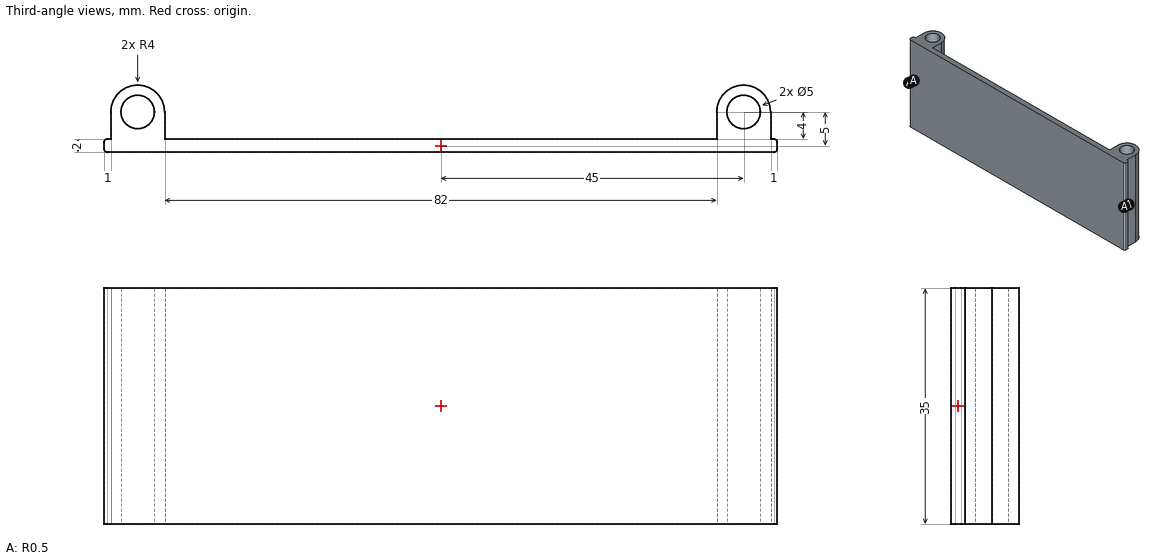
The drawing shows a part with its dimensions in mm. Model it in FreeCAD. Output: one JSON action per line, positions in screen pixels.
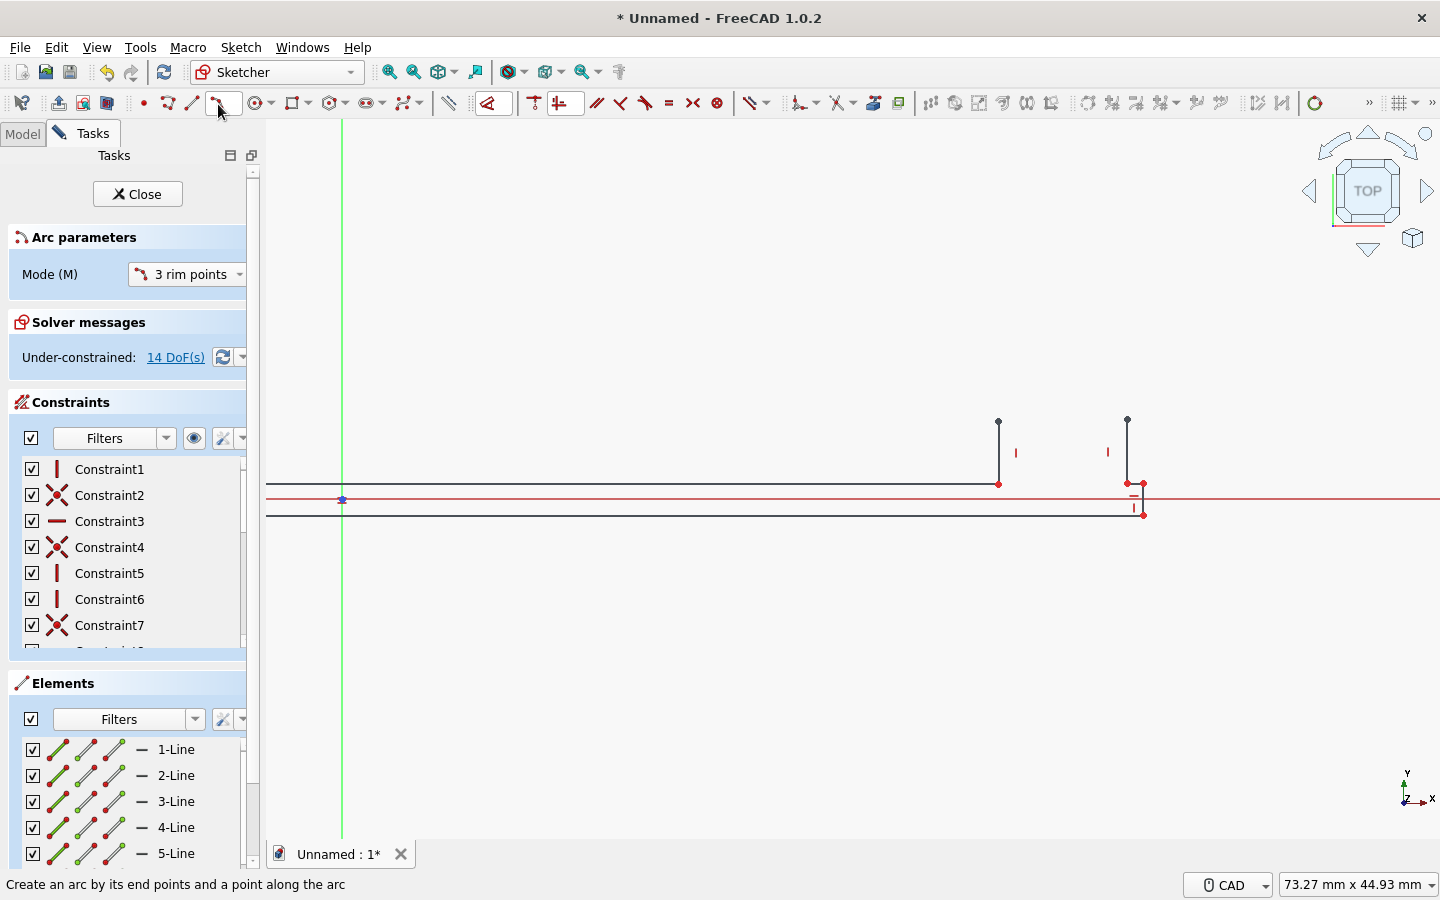
{"action": "scroll", "coordinate": [1145, 515], "scroll_direction": "down", "scroll_amount": 4}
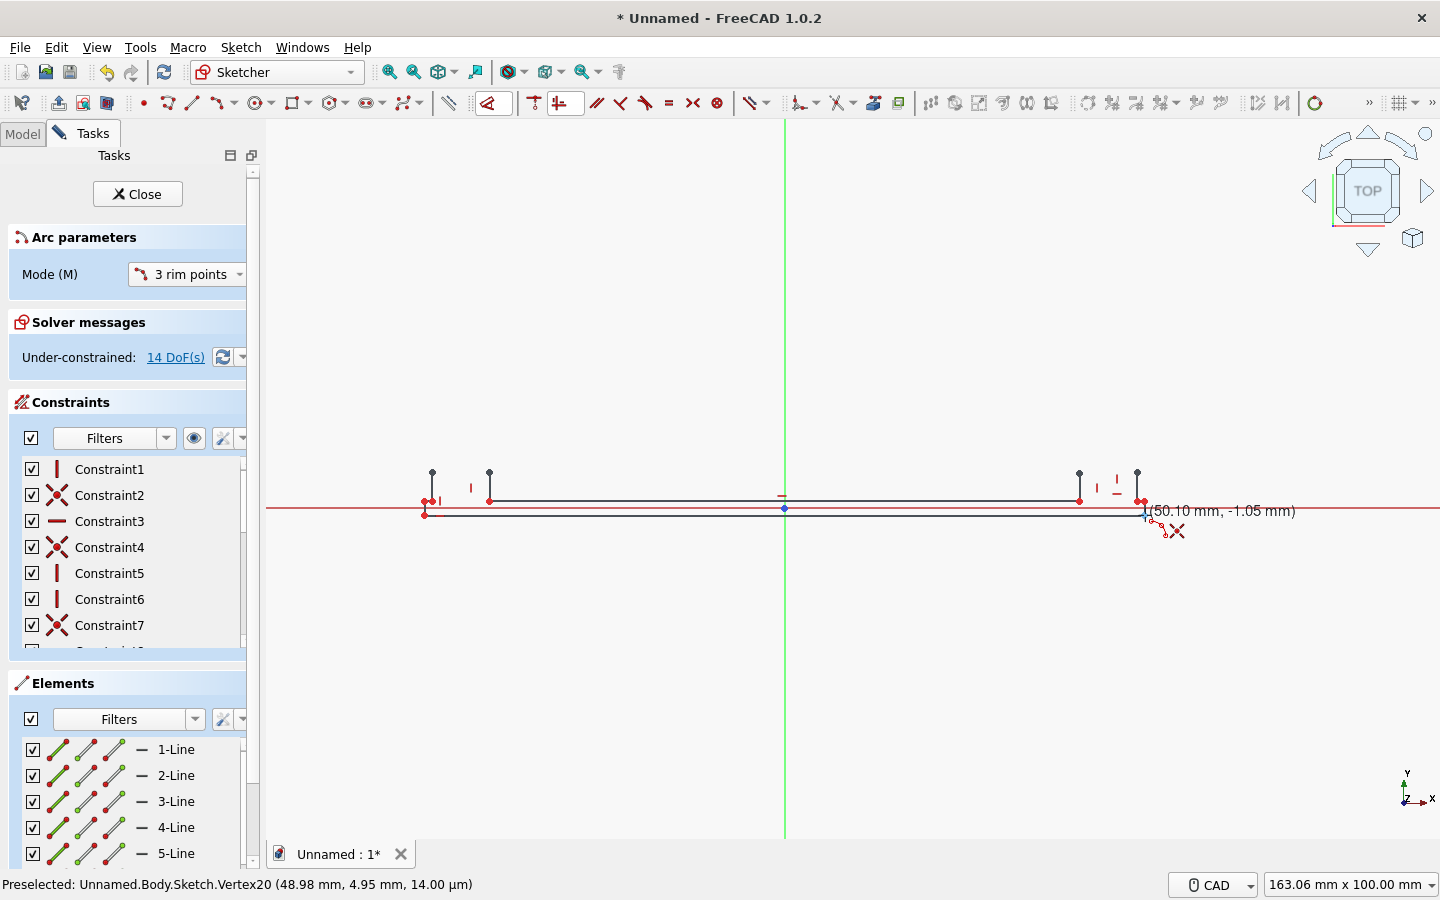
{"action": "left_click", "coordinate": [490, 473]}
{"action": "left_click", "coordinate": [432, 473]}
{"action": "left_click", "coordinate": [461, 443]}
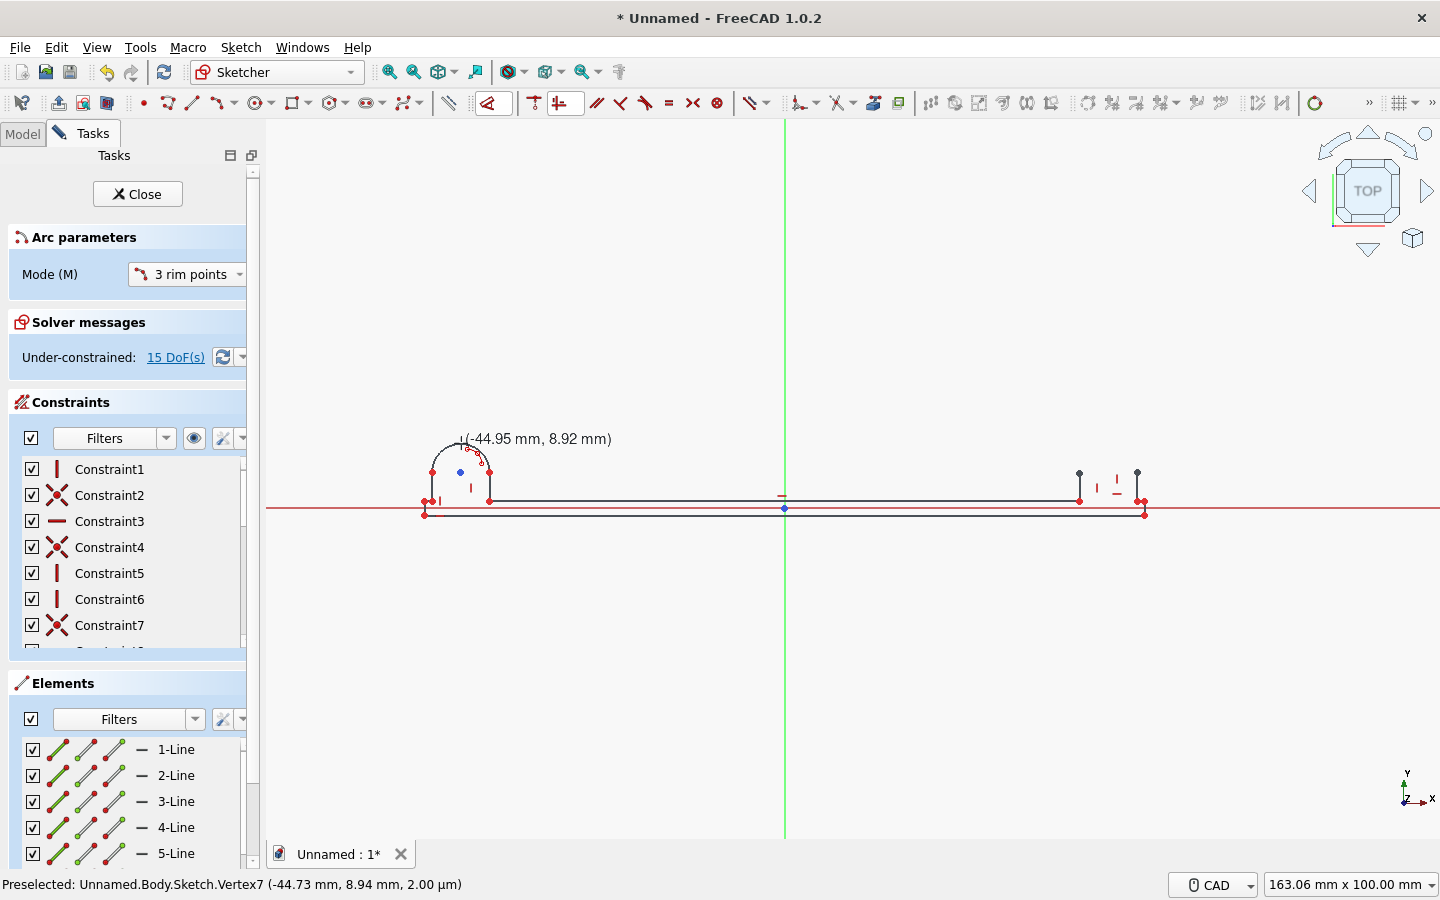
{"action": "left_click", "coordinate": [1137, 473]}
{"action": "left_click", "coordinate": [1080, 473]}
{"action": "left_click", "coordinate": [1109, 443]}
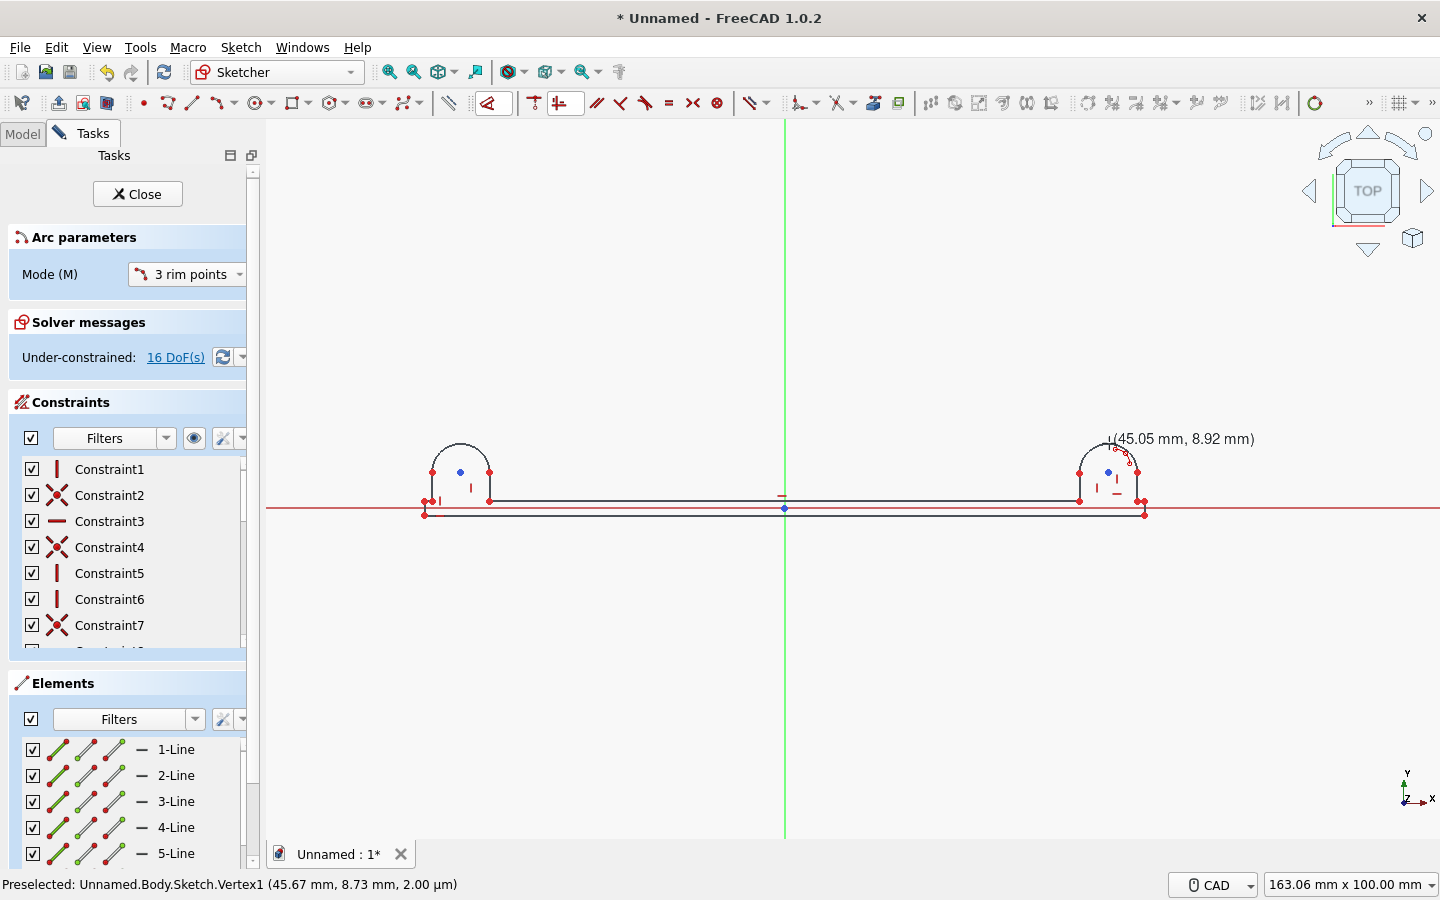
{"action": "left_click", "coordinate": [256, 104]}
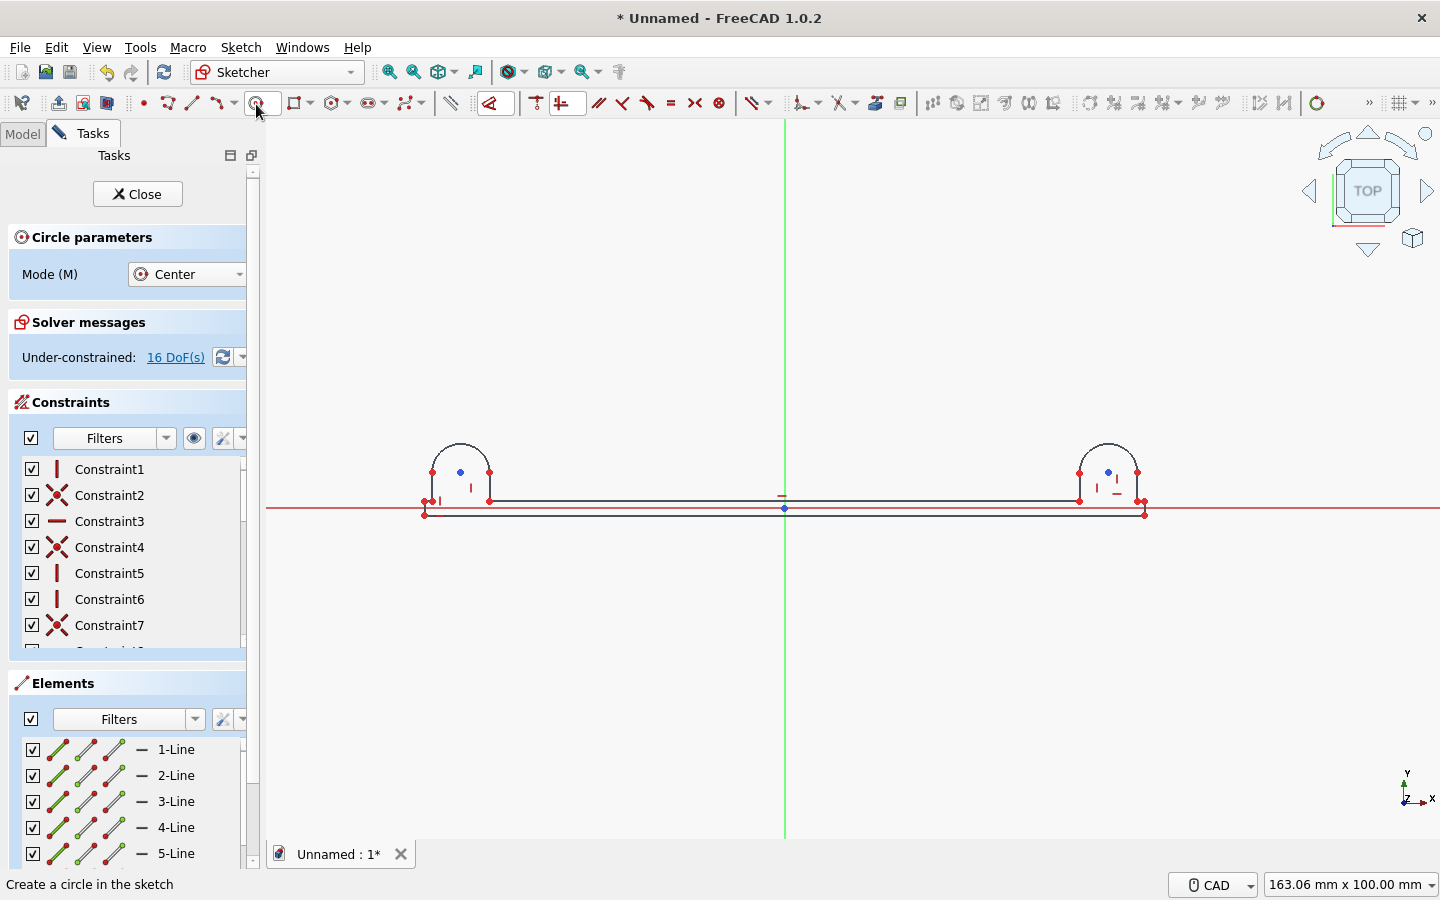
{"action": "scroll", "coordinate": [1109, 472], "scroll_direction": "up", "scroll_amount": 2}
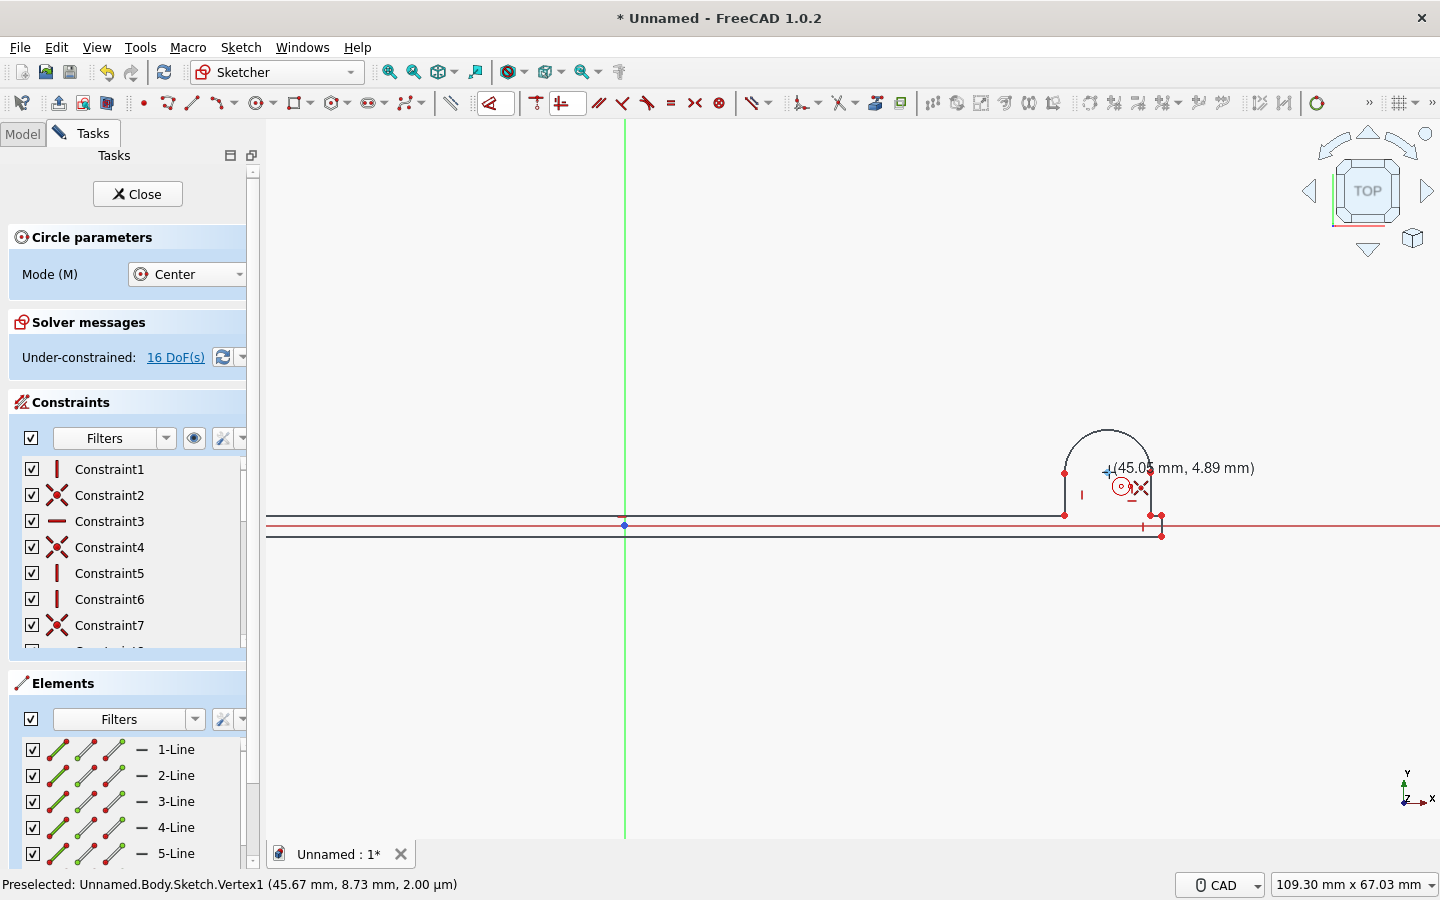
{"action": "left_click", "coordinate": [1108, 472]}
{"action": "mouse_move", "coordinate": [1127, 453]}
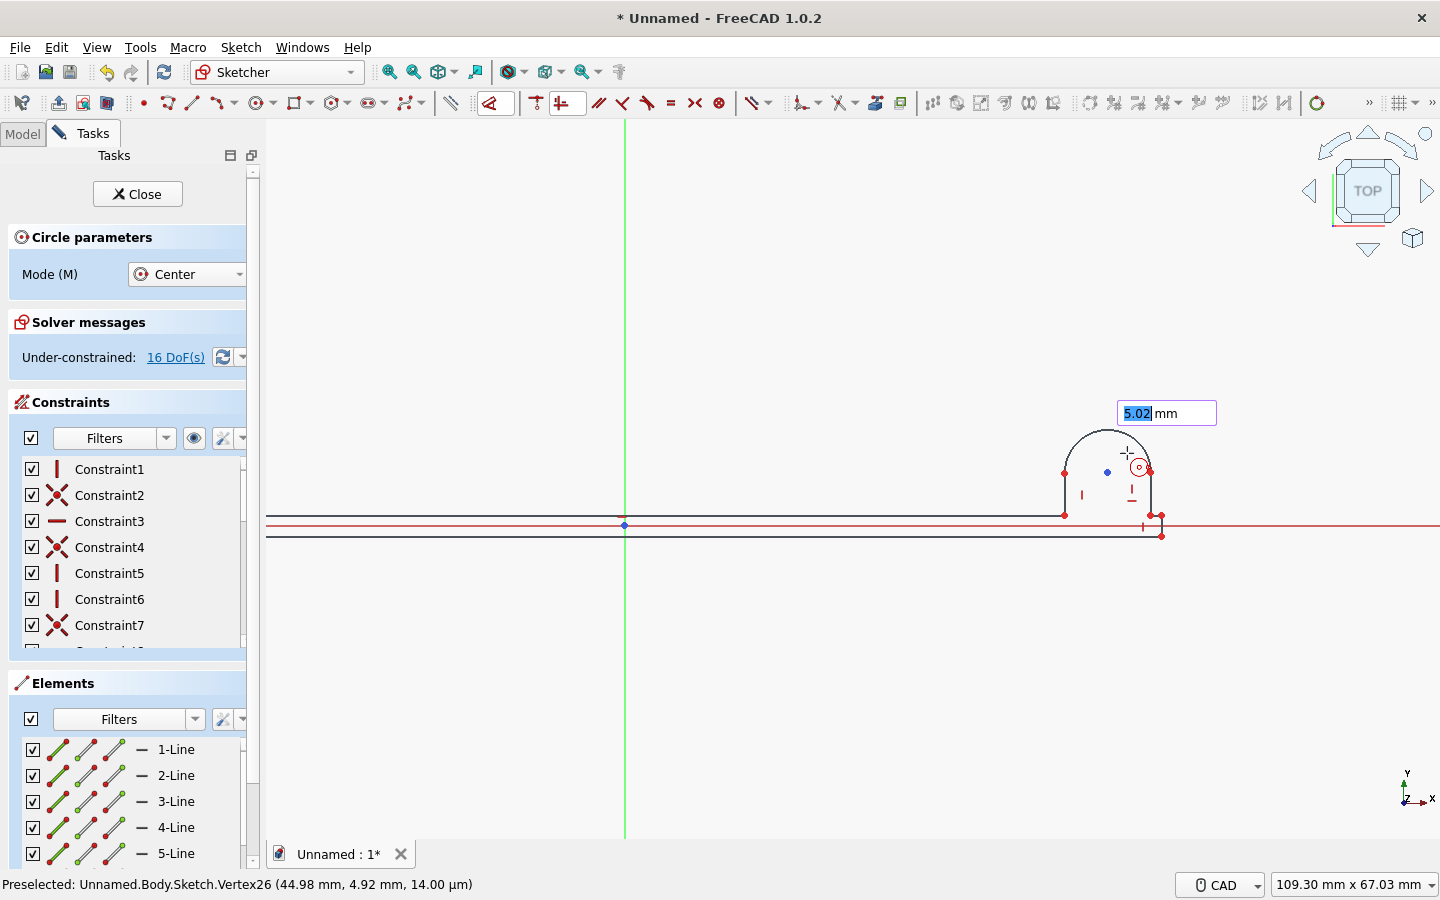
{"action": "type", "text": "5"}
{"action": "key", "text": "Return"}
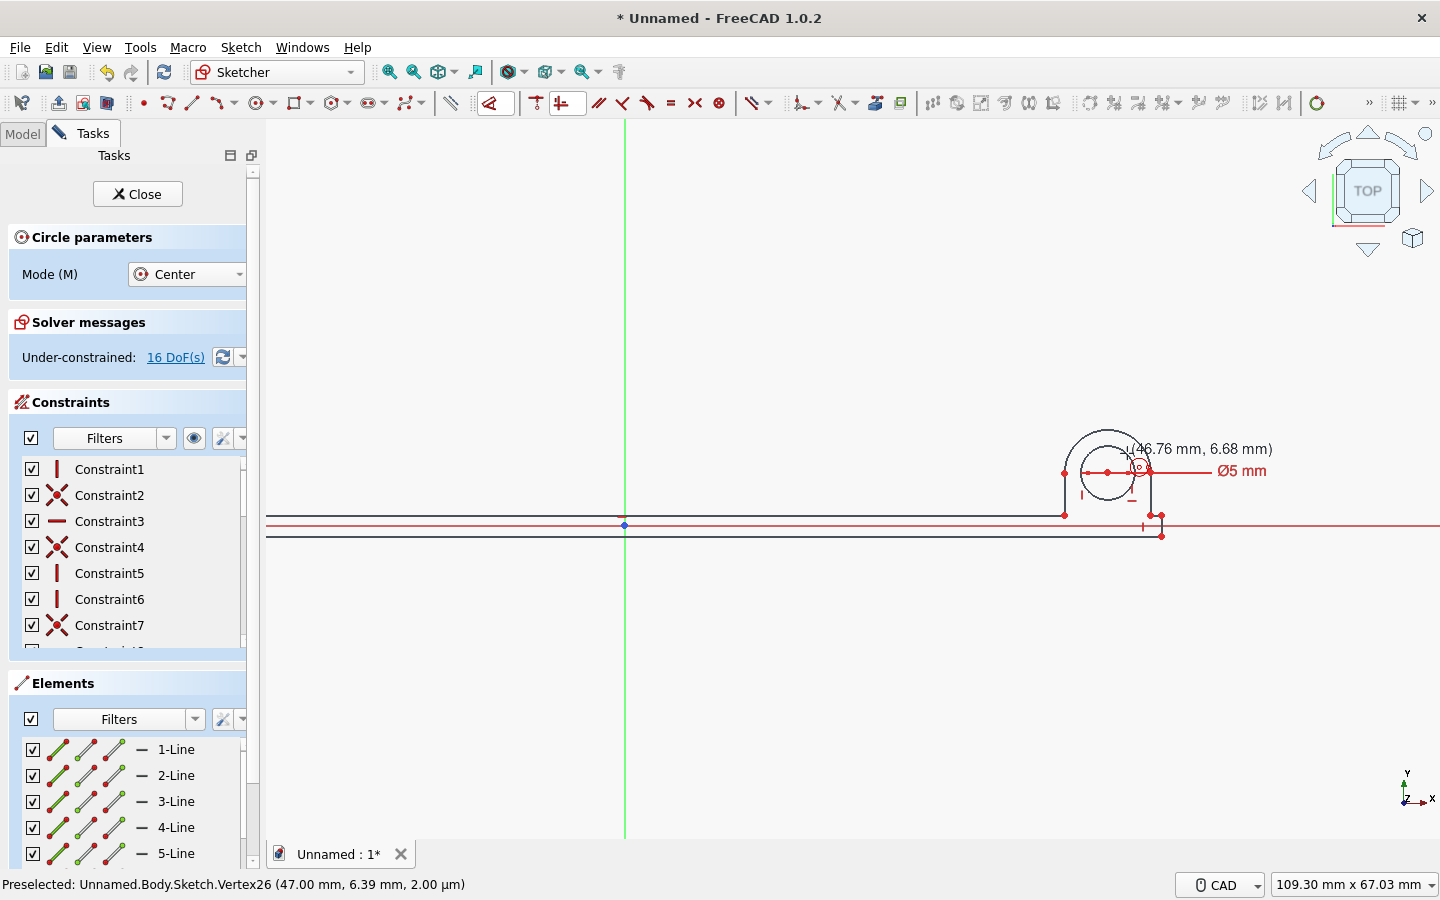
{"action": "scroll", "coordinate": [1109, 471], "scroll_direction": "down", "scroll_amount": 2}